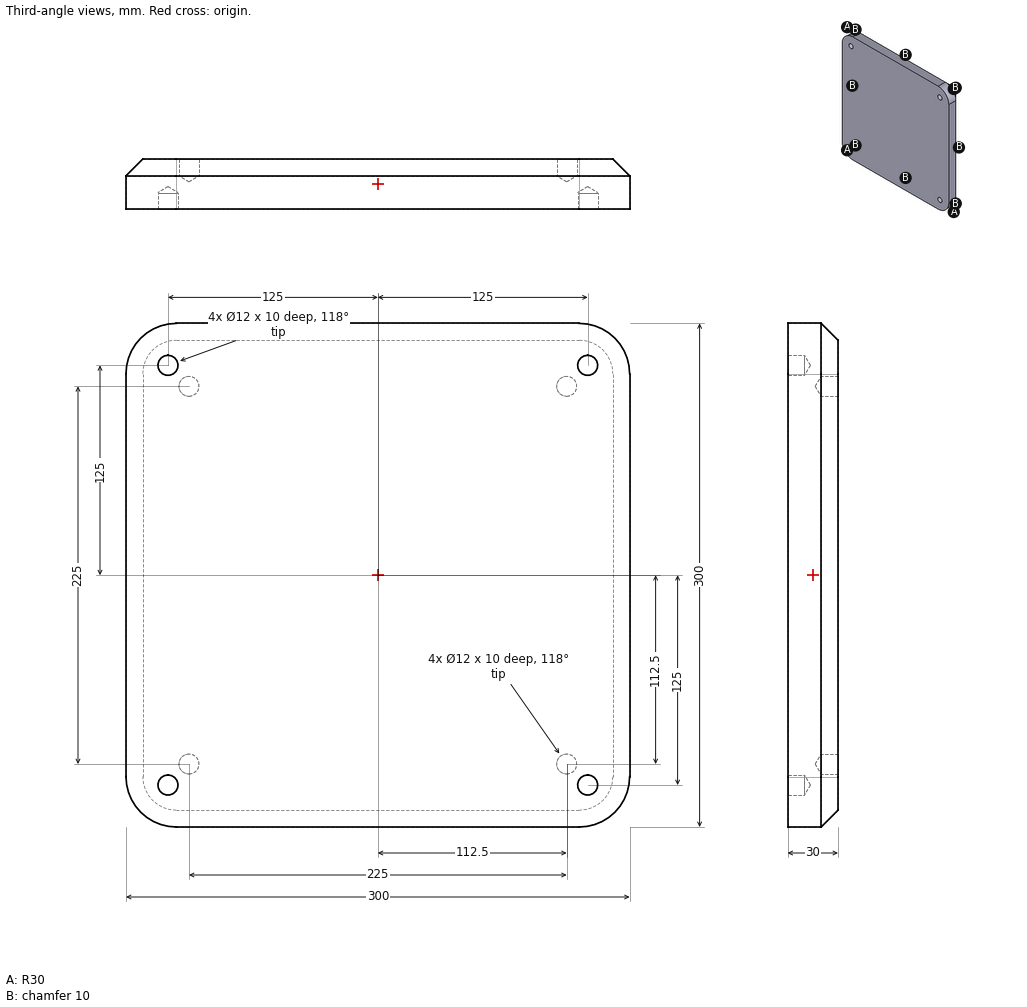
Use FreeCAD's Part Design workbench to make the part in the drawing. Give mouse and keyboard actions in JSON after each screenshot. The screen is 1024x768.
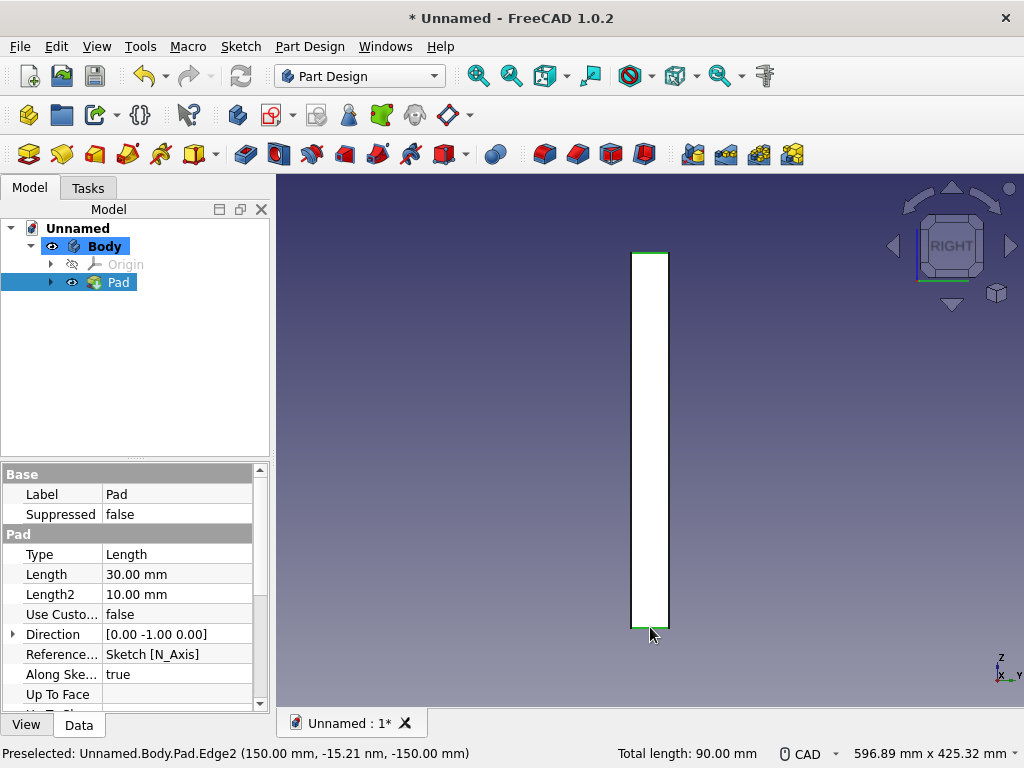
{"action": "key", "text": "5"}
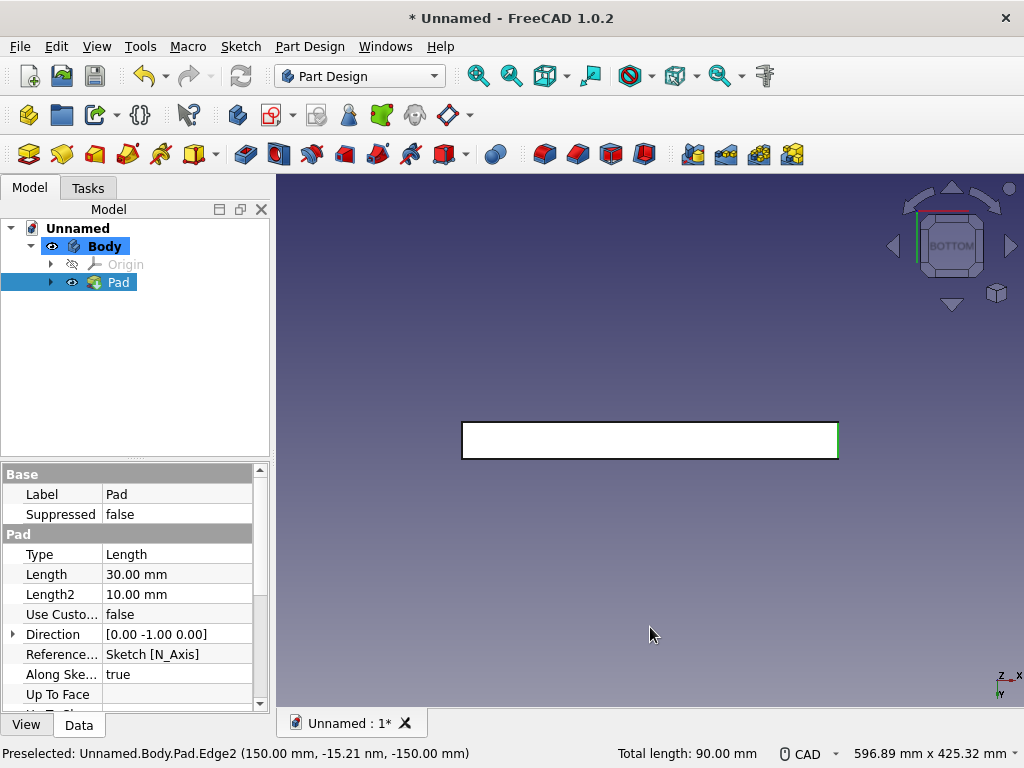
{"action": "left_click", "coordinate": [462, 440], "text": "ctrl"}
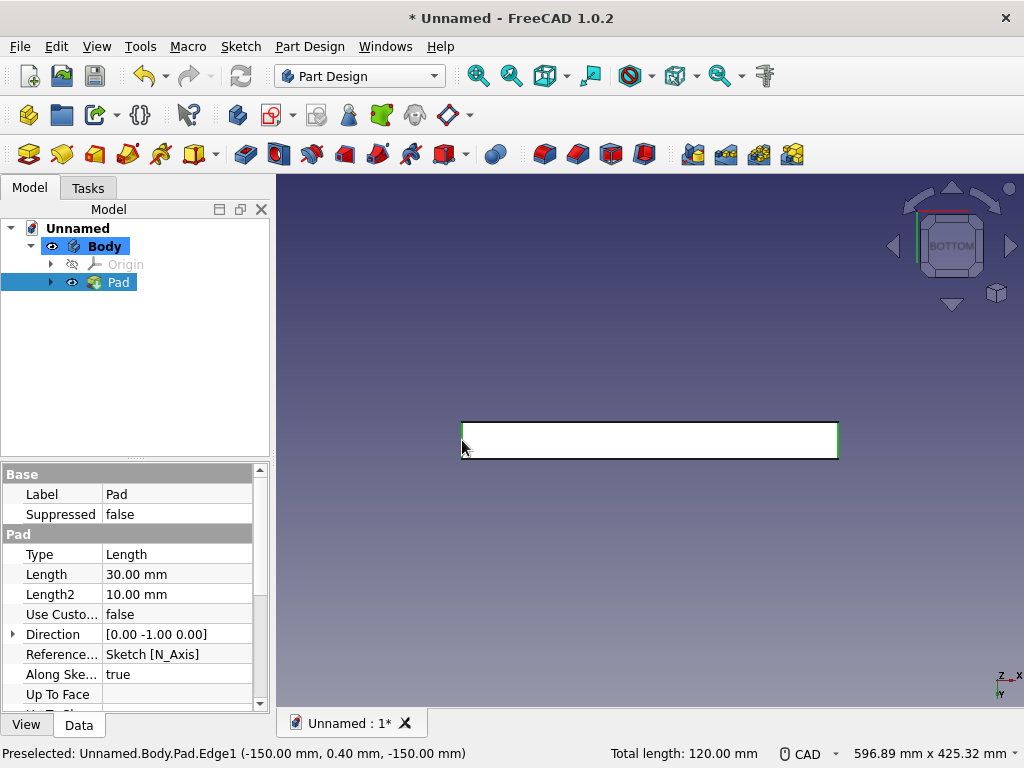
{"action": "left_click", "coordinate": [545, 154]}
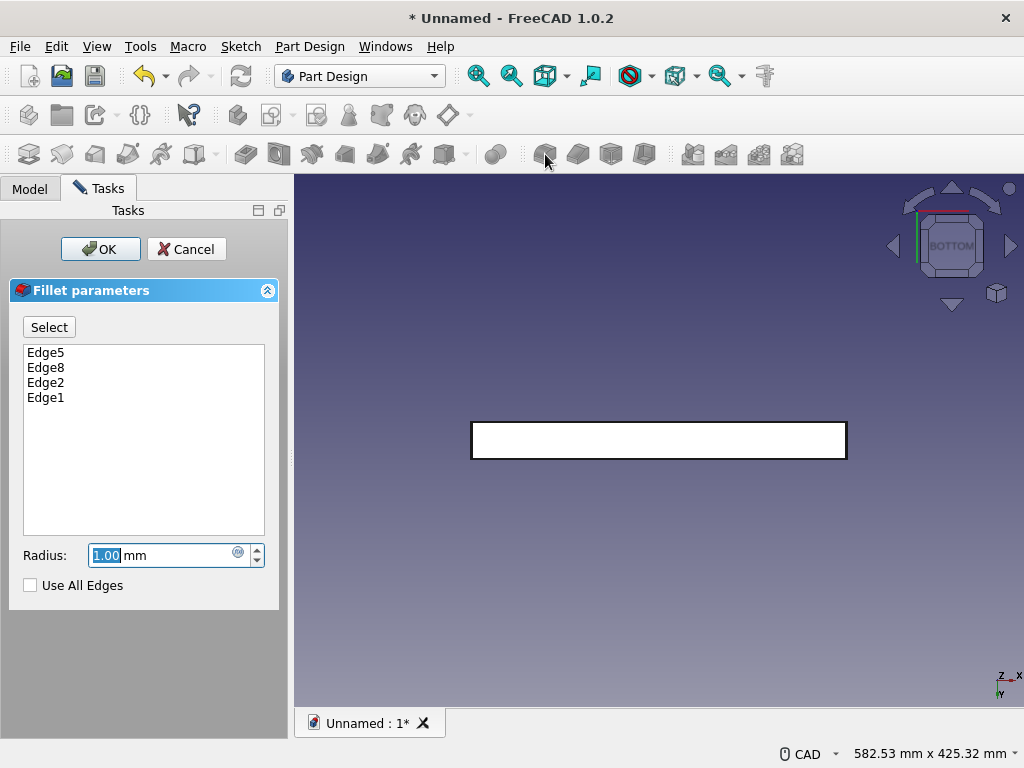
{"action": "type", "text": "30"}
{"action": "key", "text": "Tab"}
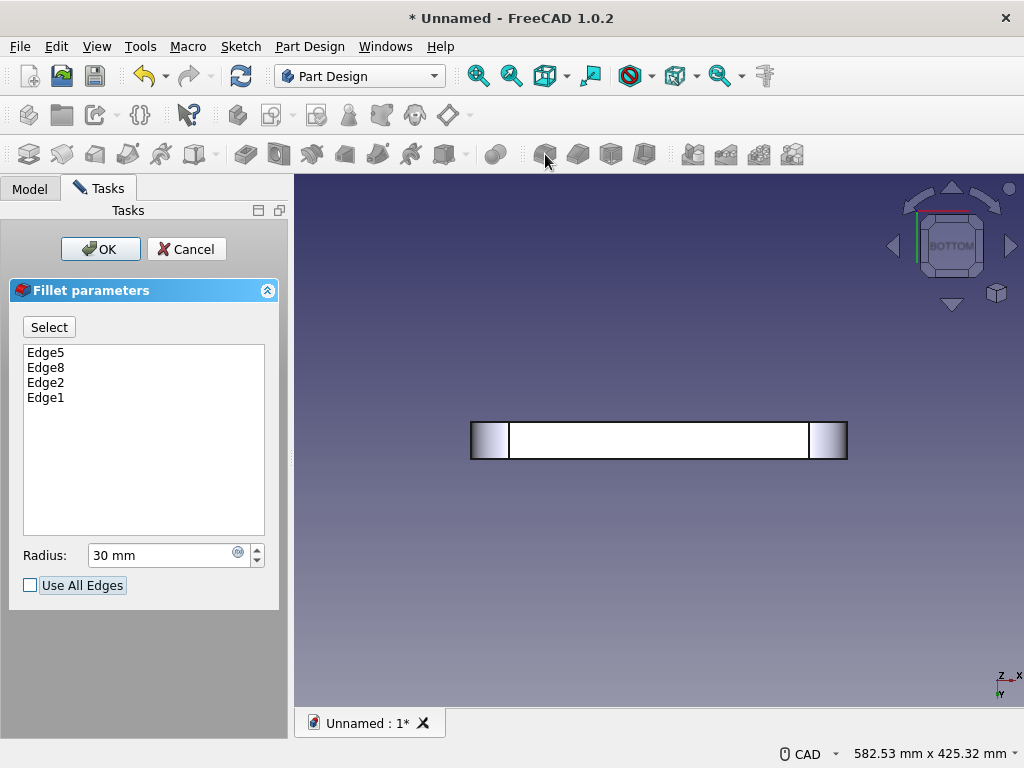
{"action": "left_click", "coordinate": [101, 249]}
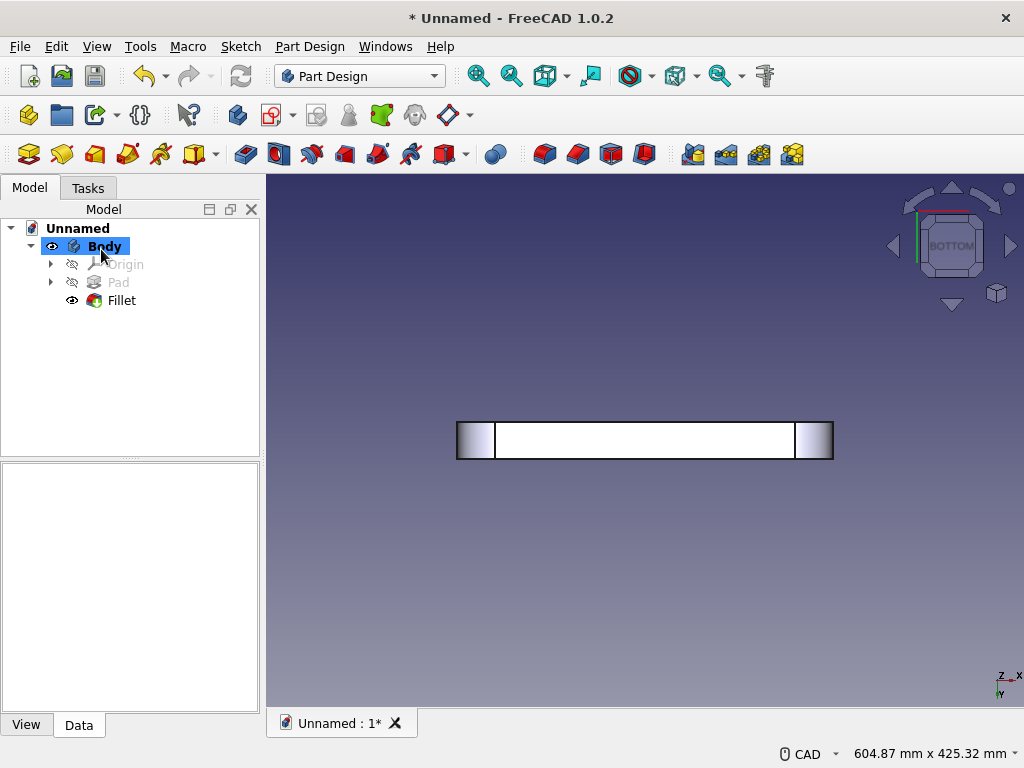
{"action": "key", "text": "0"}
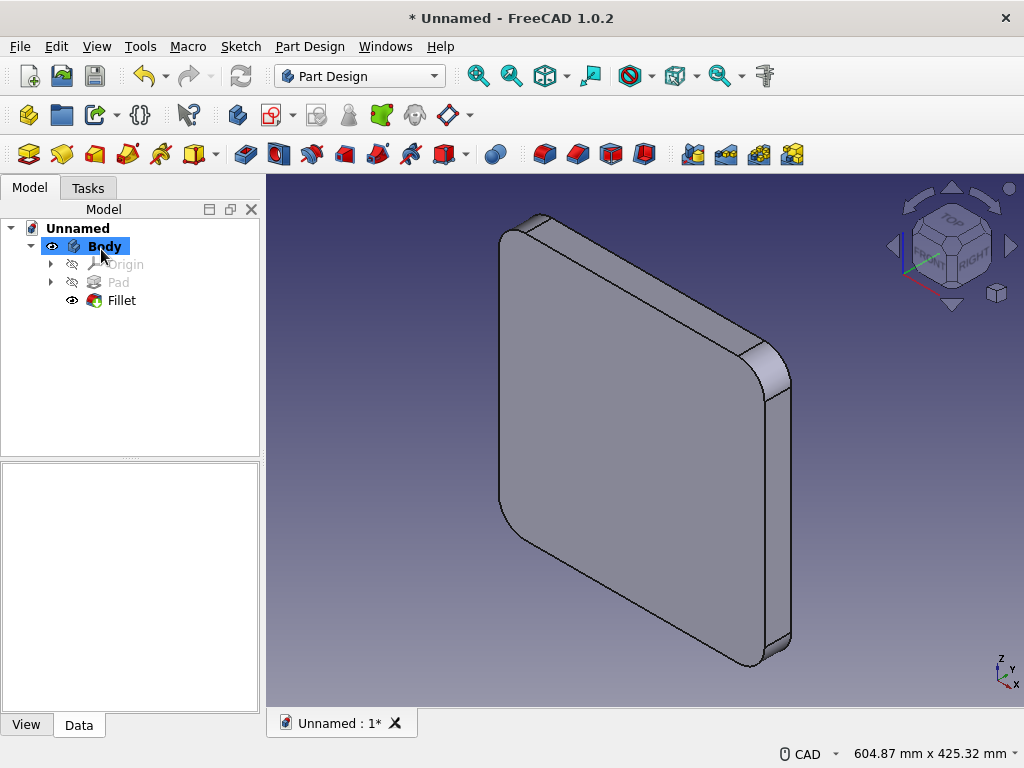
{"action": "key", "text": "2"}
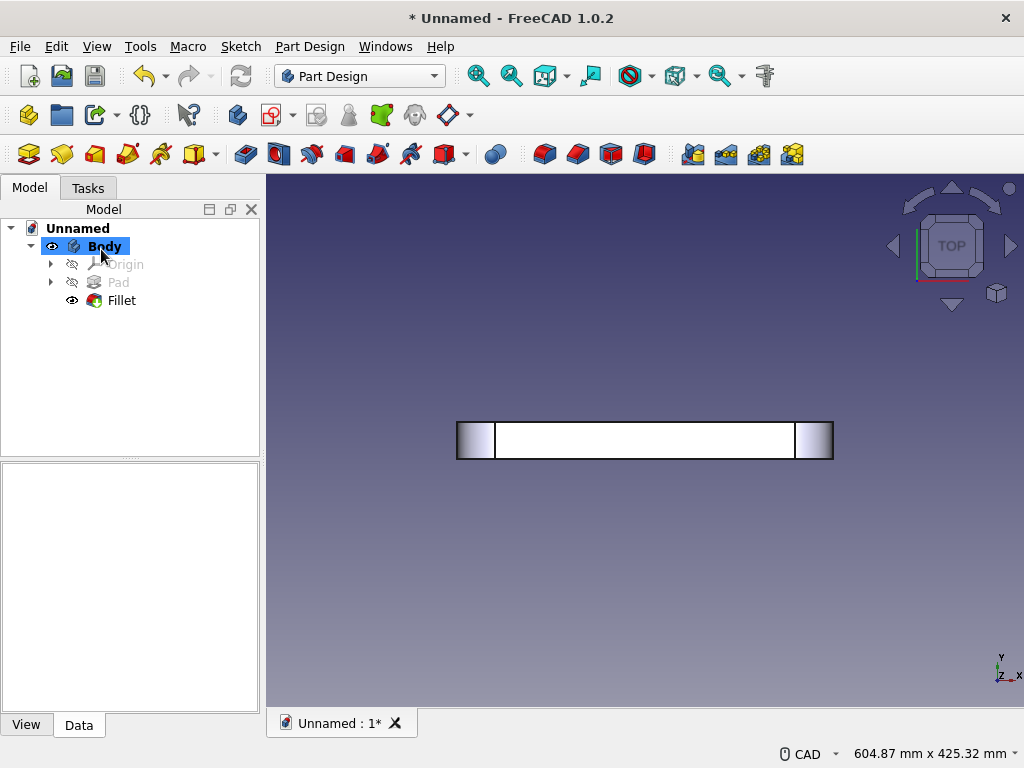
{"action": "key", "text": "1"}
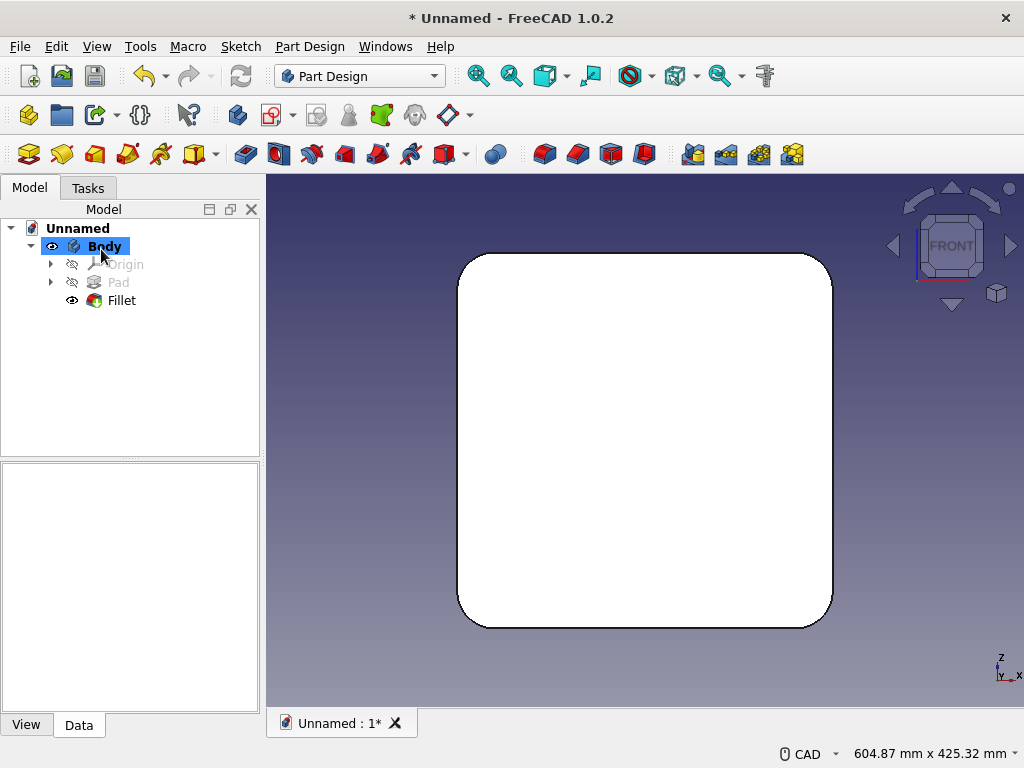
{"action": "key", "text": "3"}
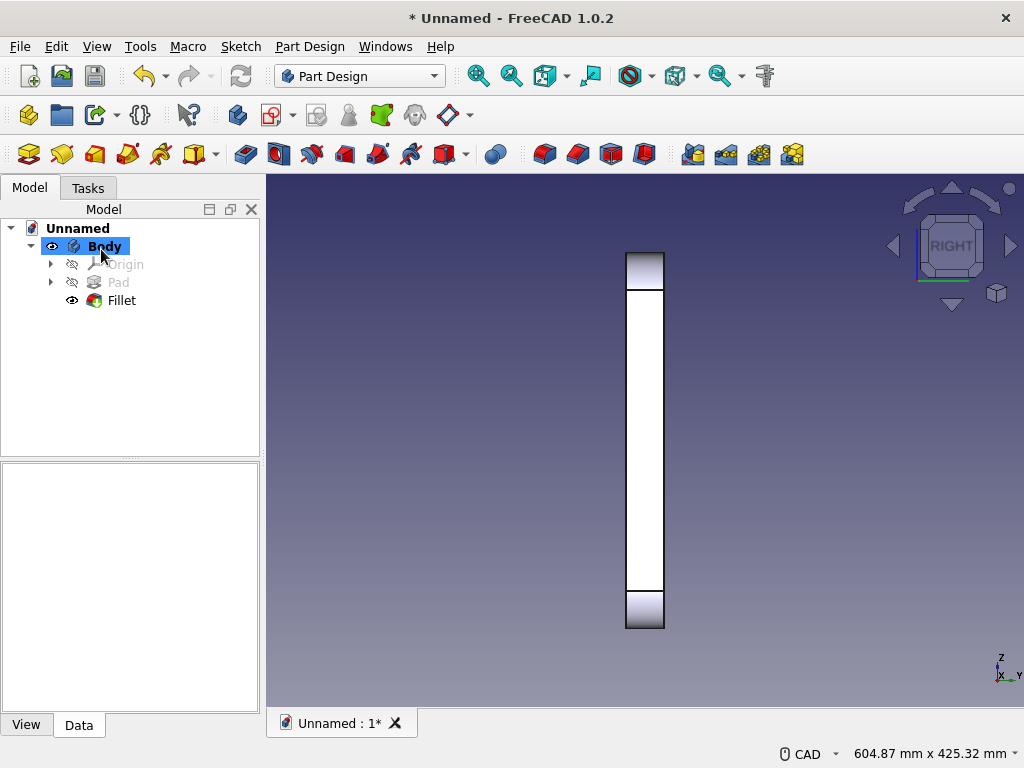
{"action": "key", "text": "5"}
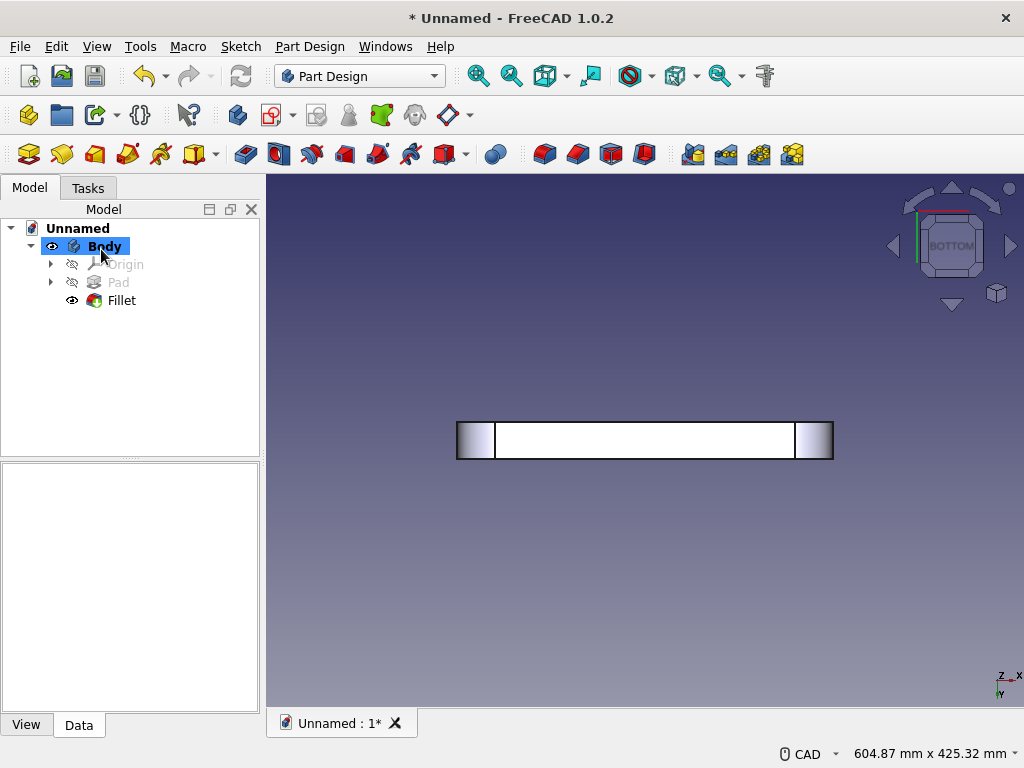
{"action": "key", "text": "4"}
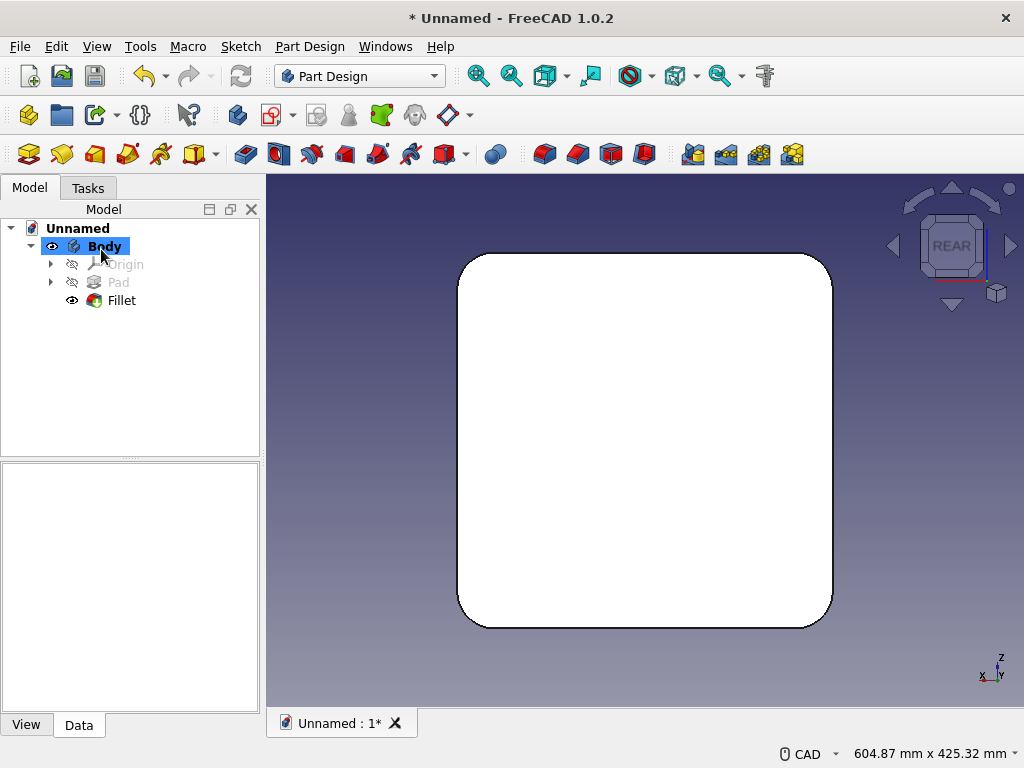
{"action": "left_click", "coordinate": [645, 439]}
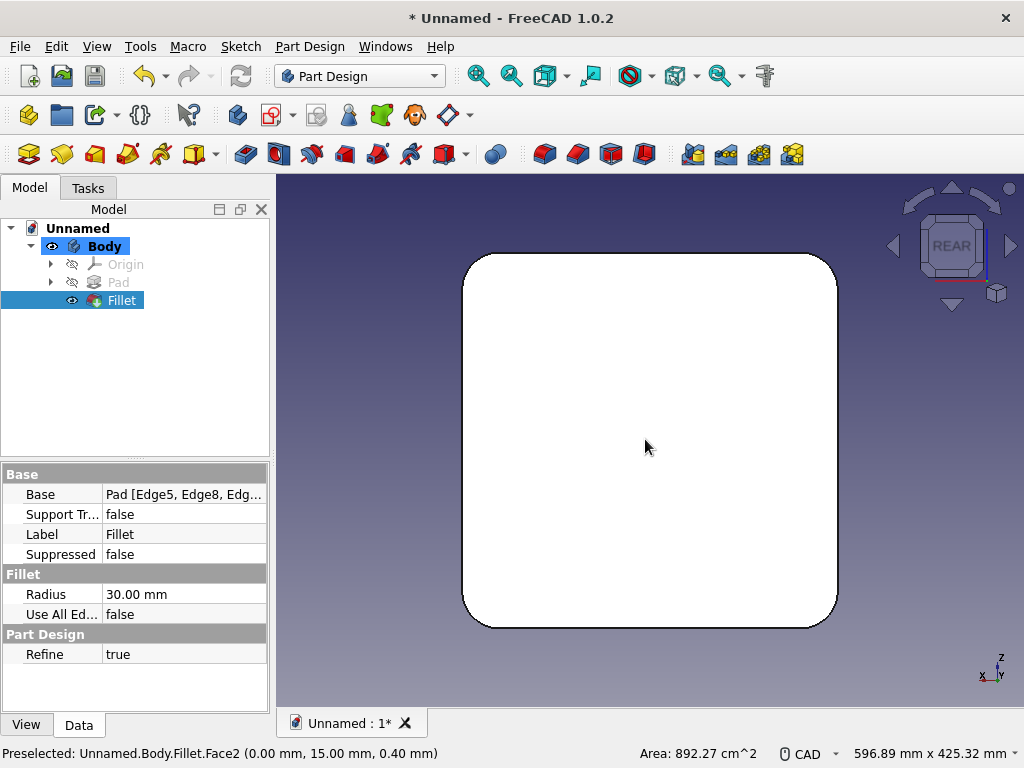
{"action": "left_click", "coordinate": [578, 154]}